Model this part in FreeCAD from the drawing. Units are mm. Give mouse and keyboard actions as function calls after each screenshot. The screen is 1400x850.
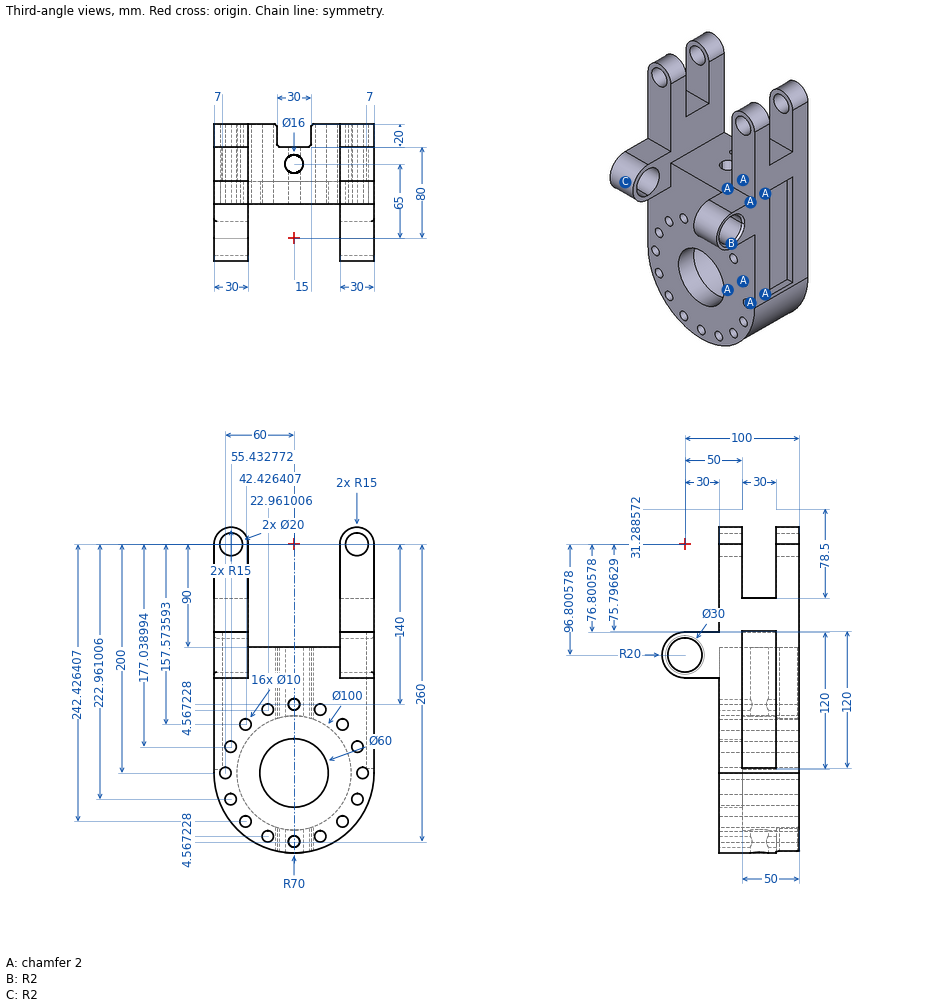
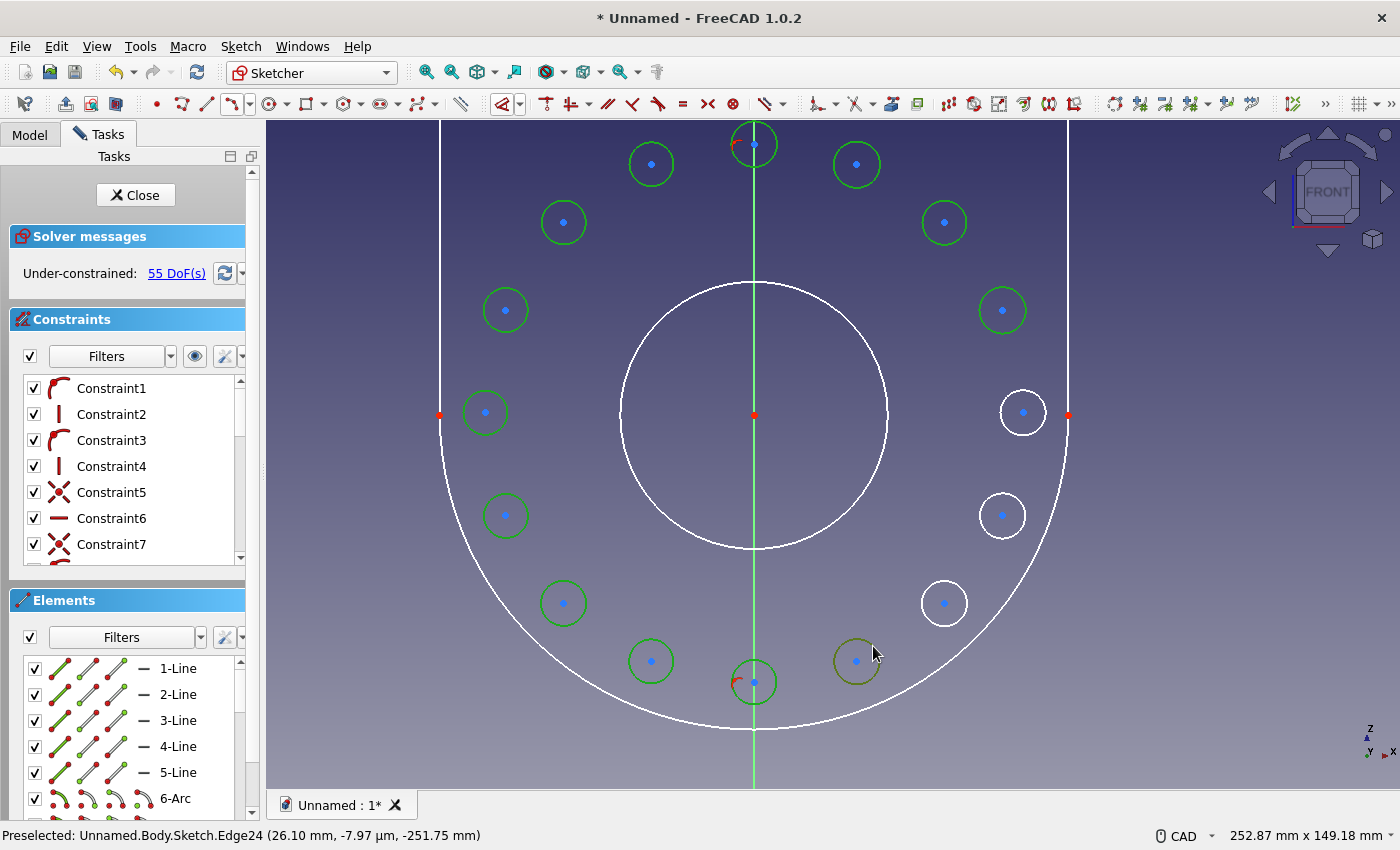
click(1039, 397)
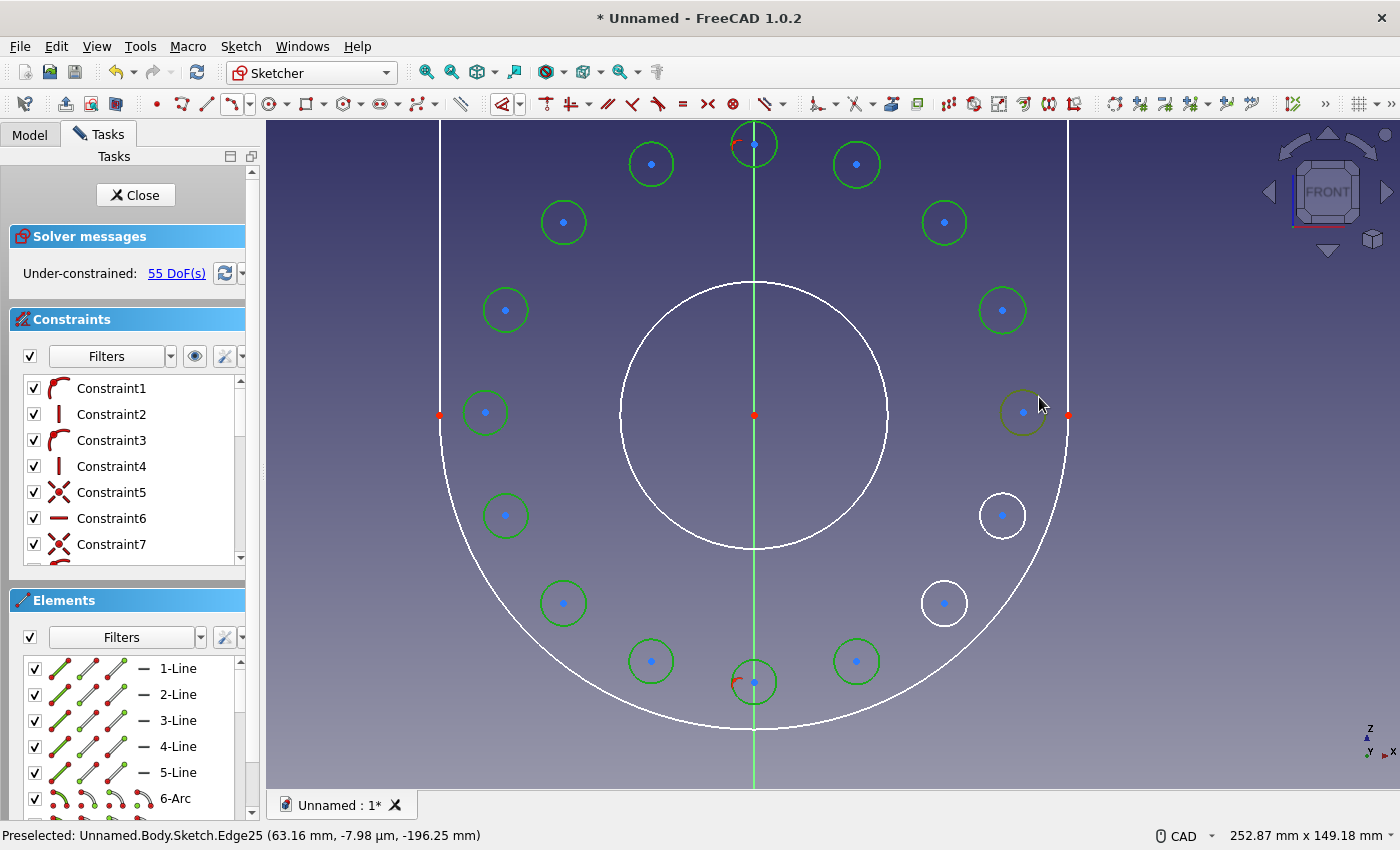
click(1019, 500)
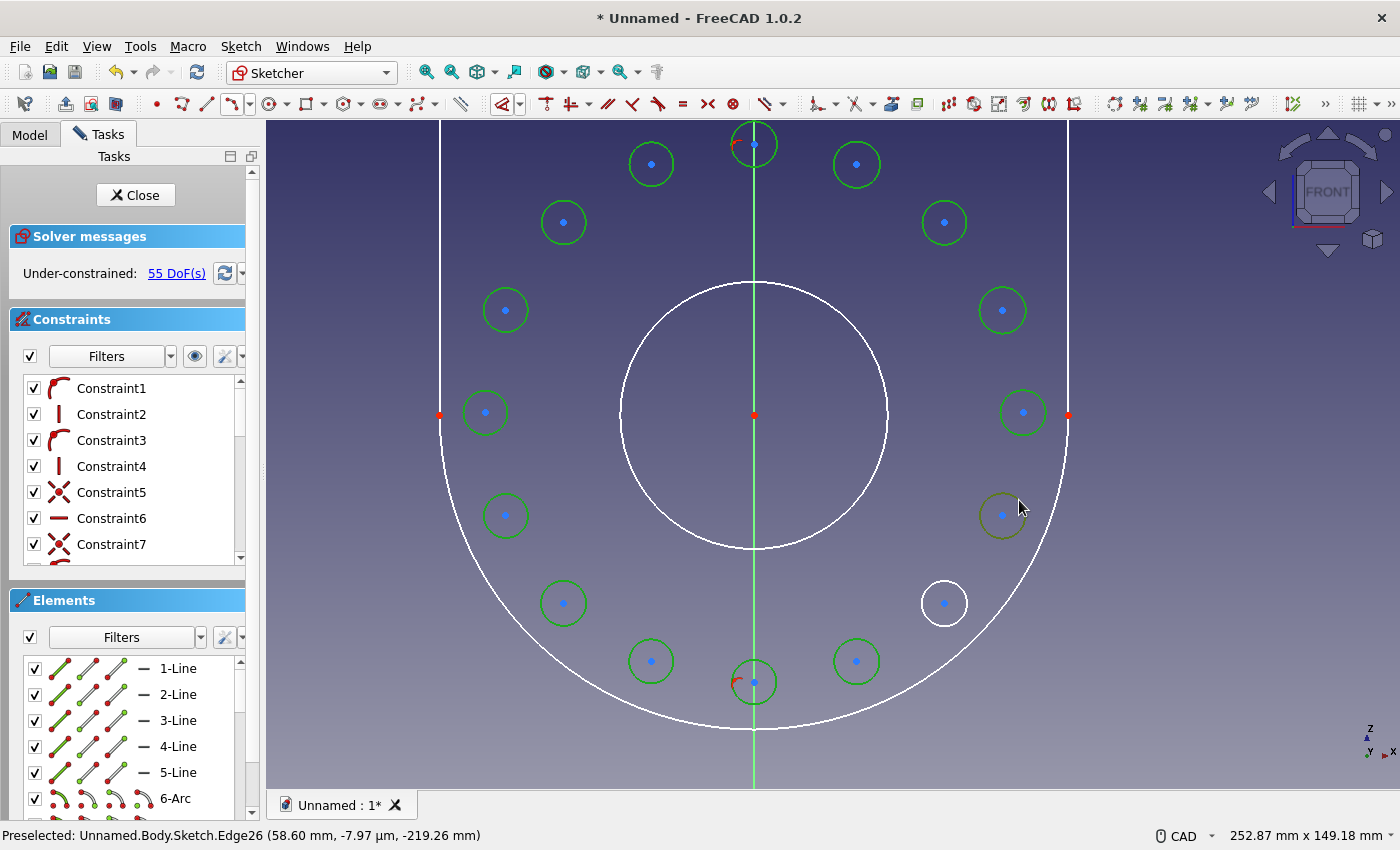
click(960, 588)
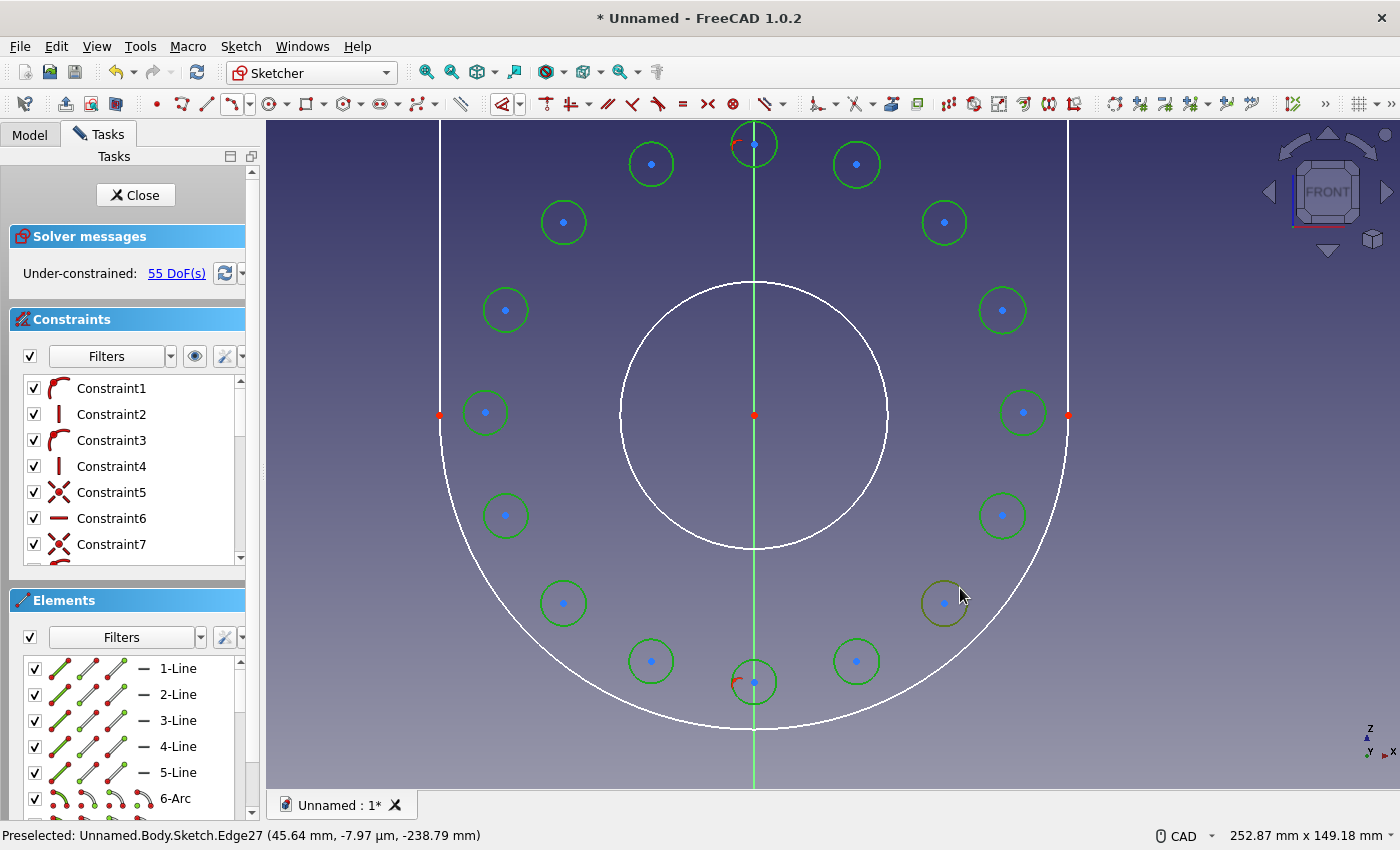
key(e)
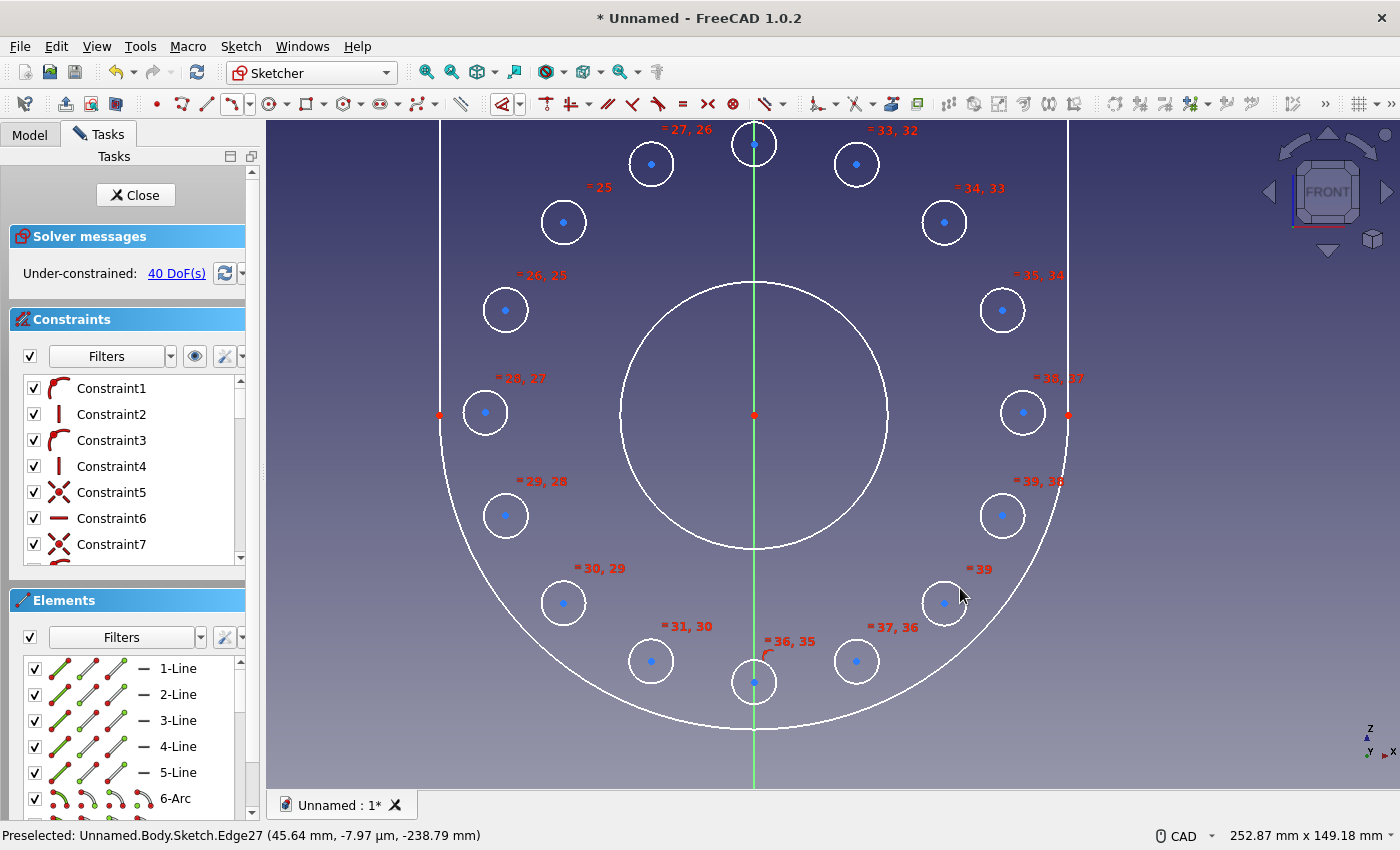
click(754, 415)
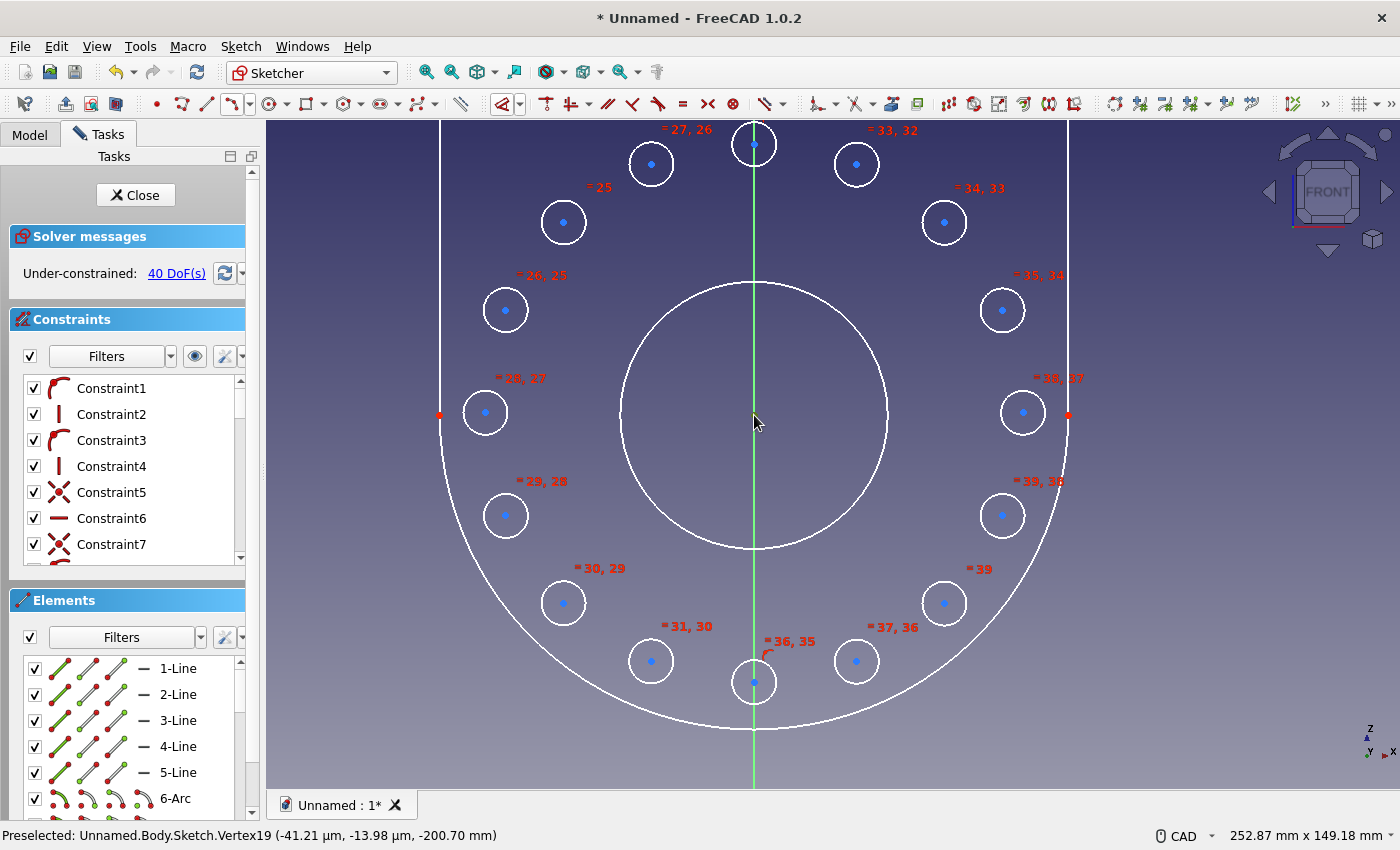
click(754, 630)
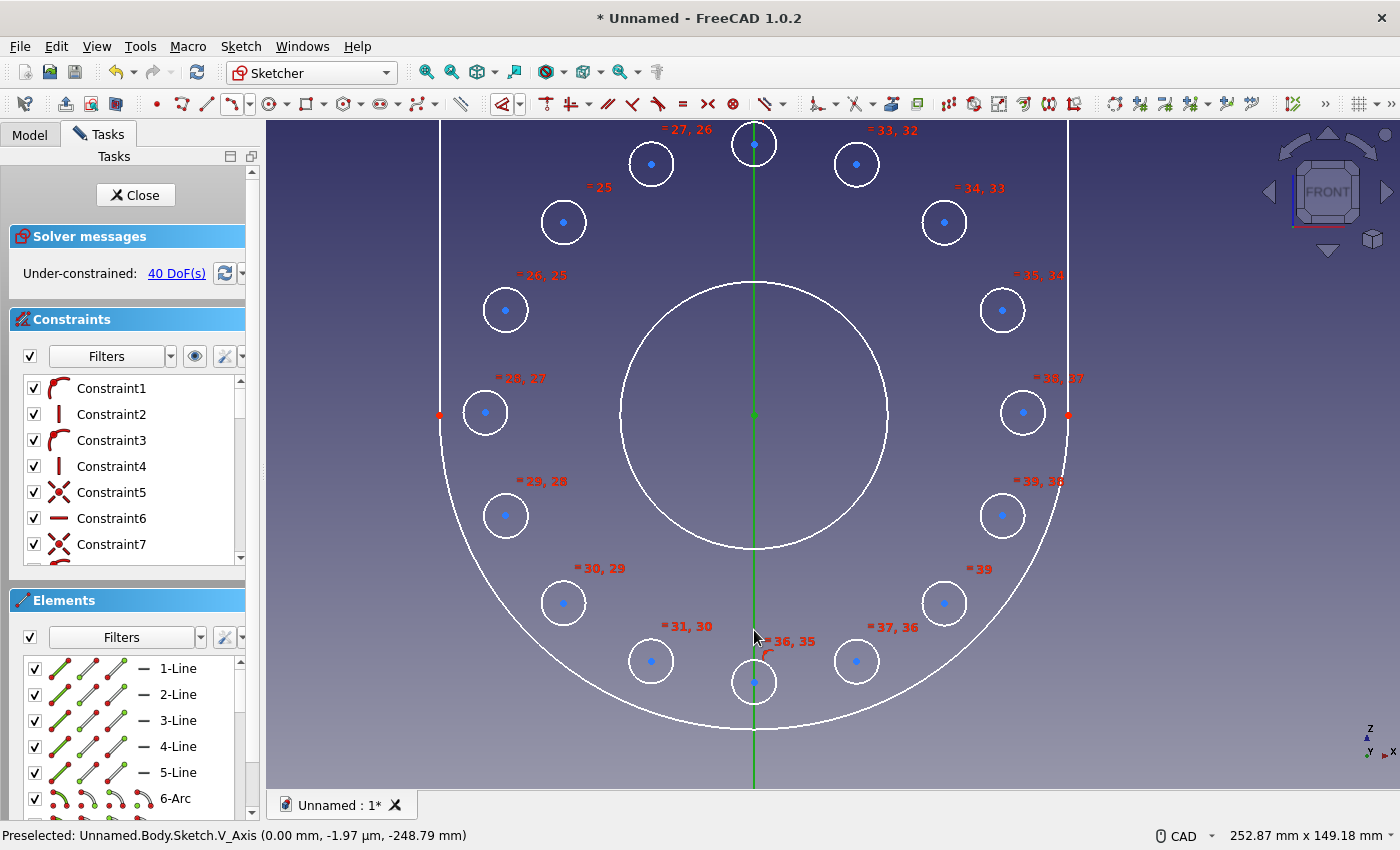
key(c)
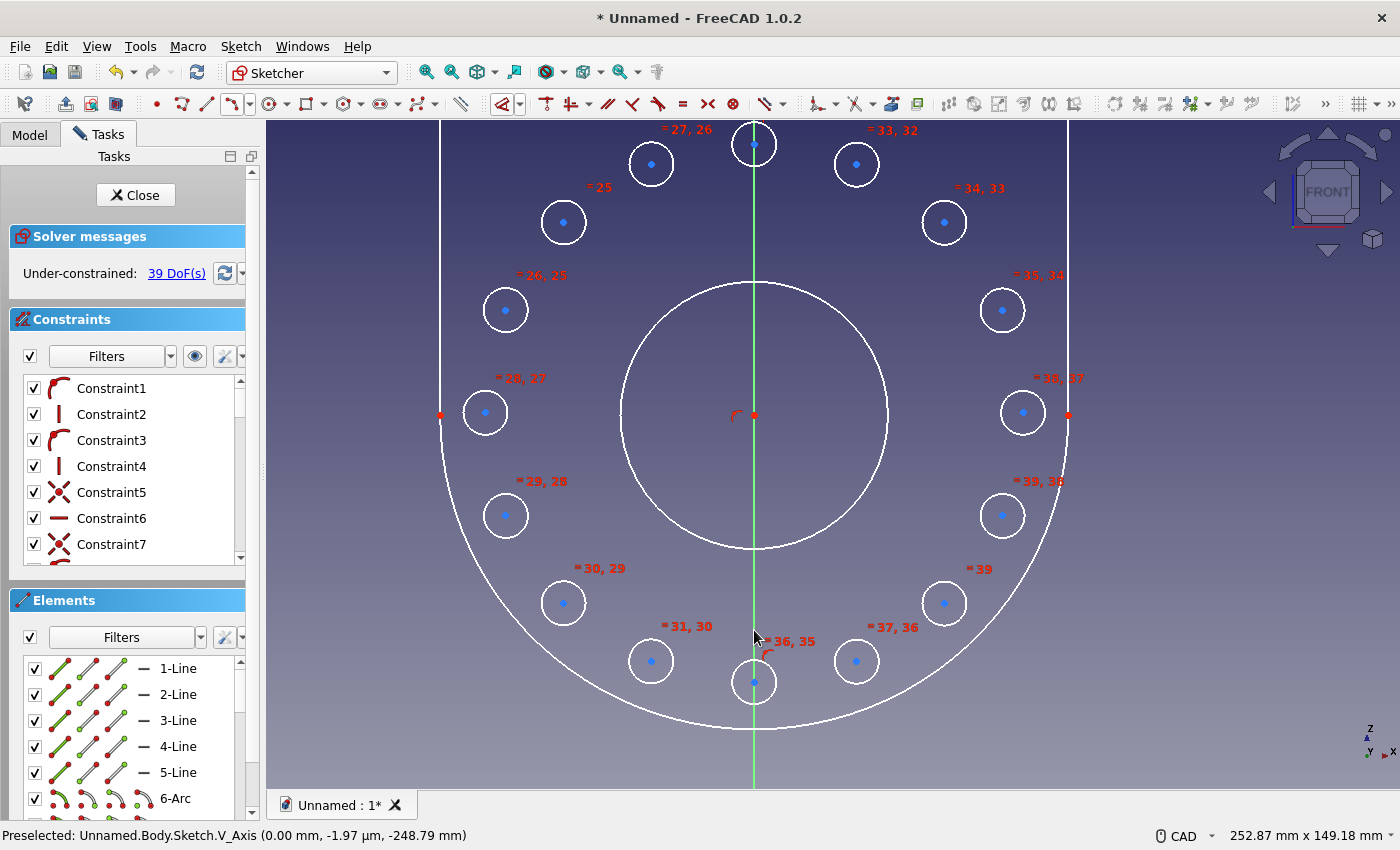
click(651, 164)